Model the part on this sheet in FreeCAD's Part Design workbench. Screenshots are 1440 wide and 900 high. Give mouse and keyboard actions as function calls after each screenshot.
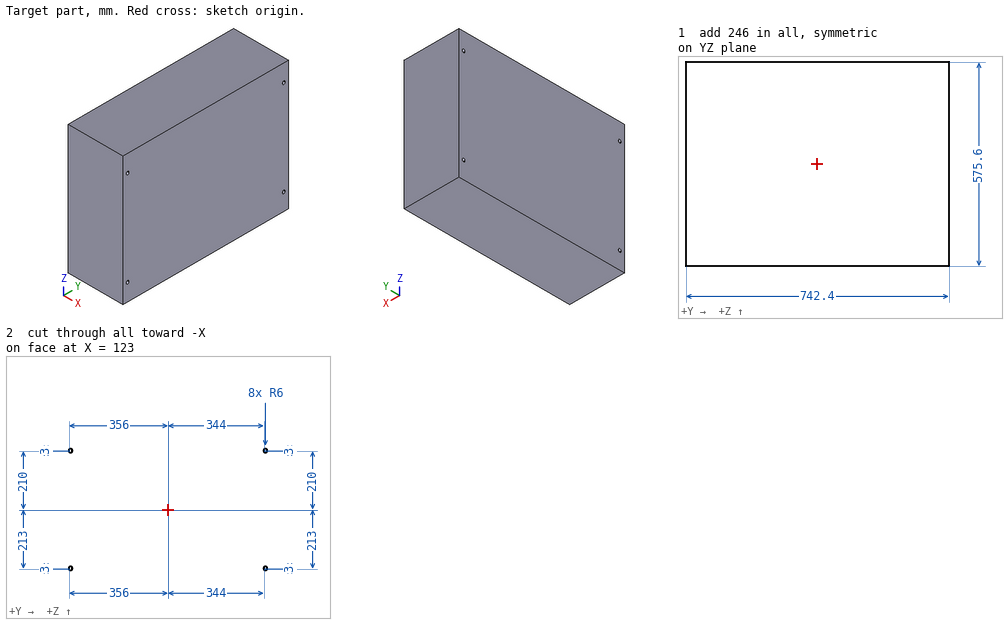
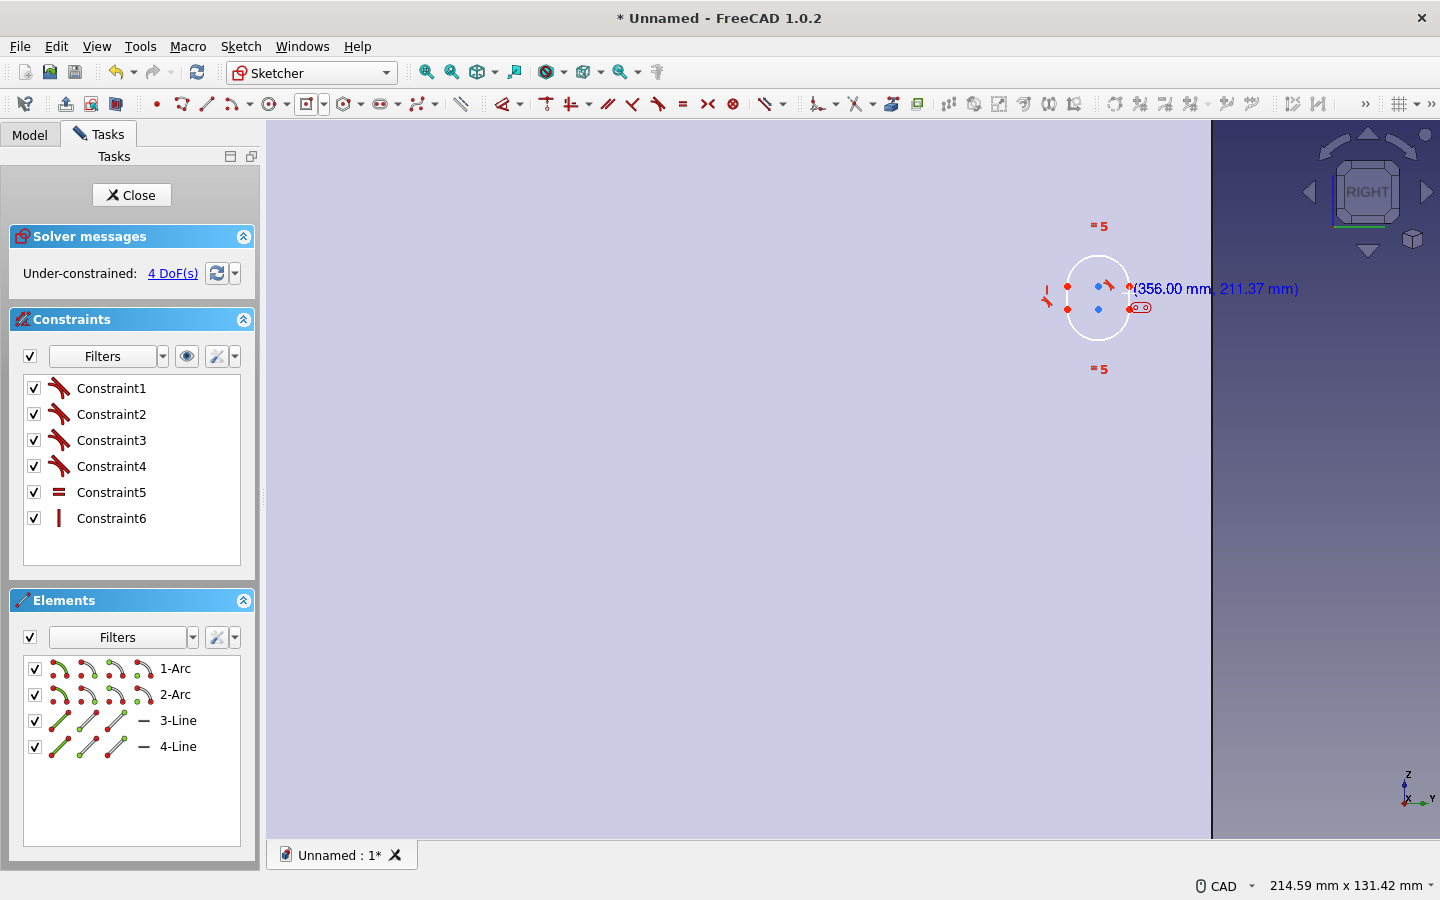
scroll(1102, 287, down, 9)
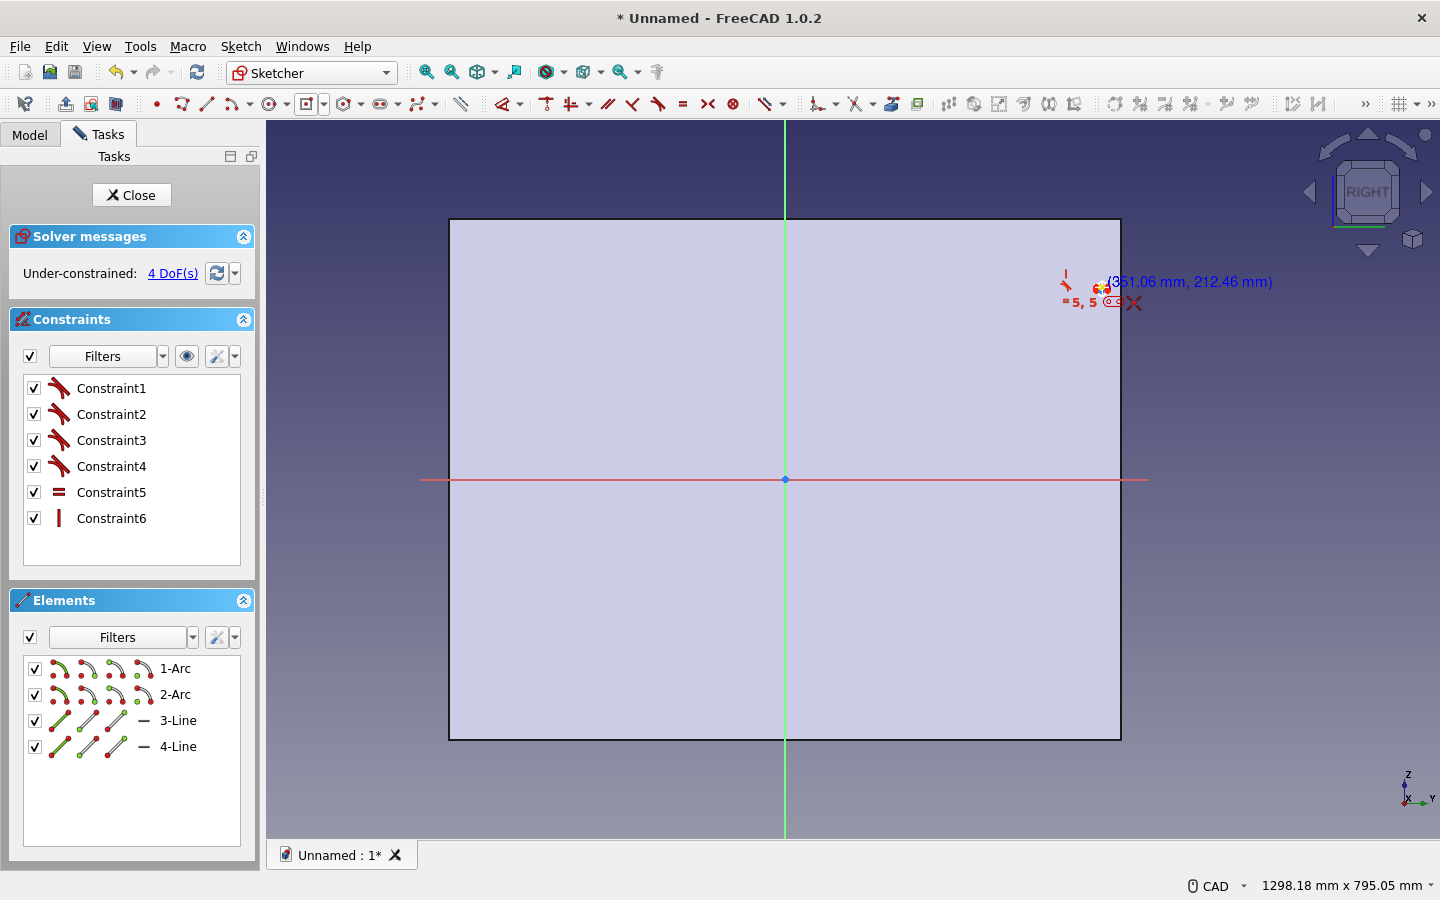
scroll(1102, 672, up, 8)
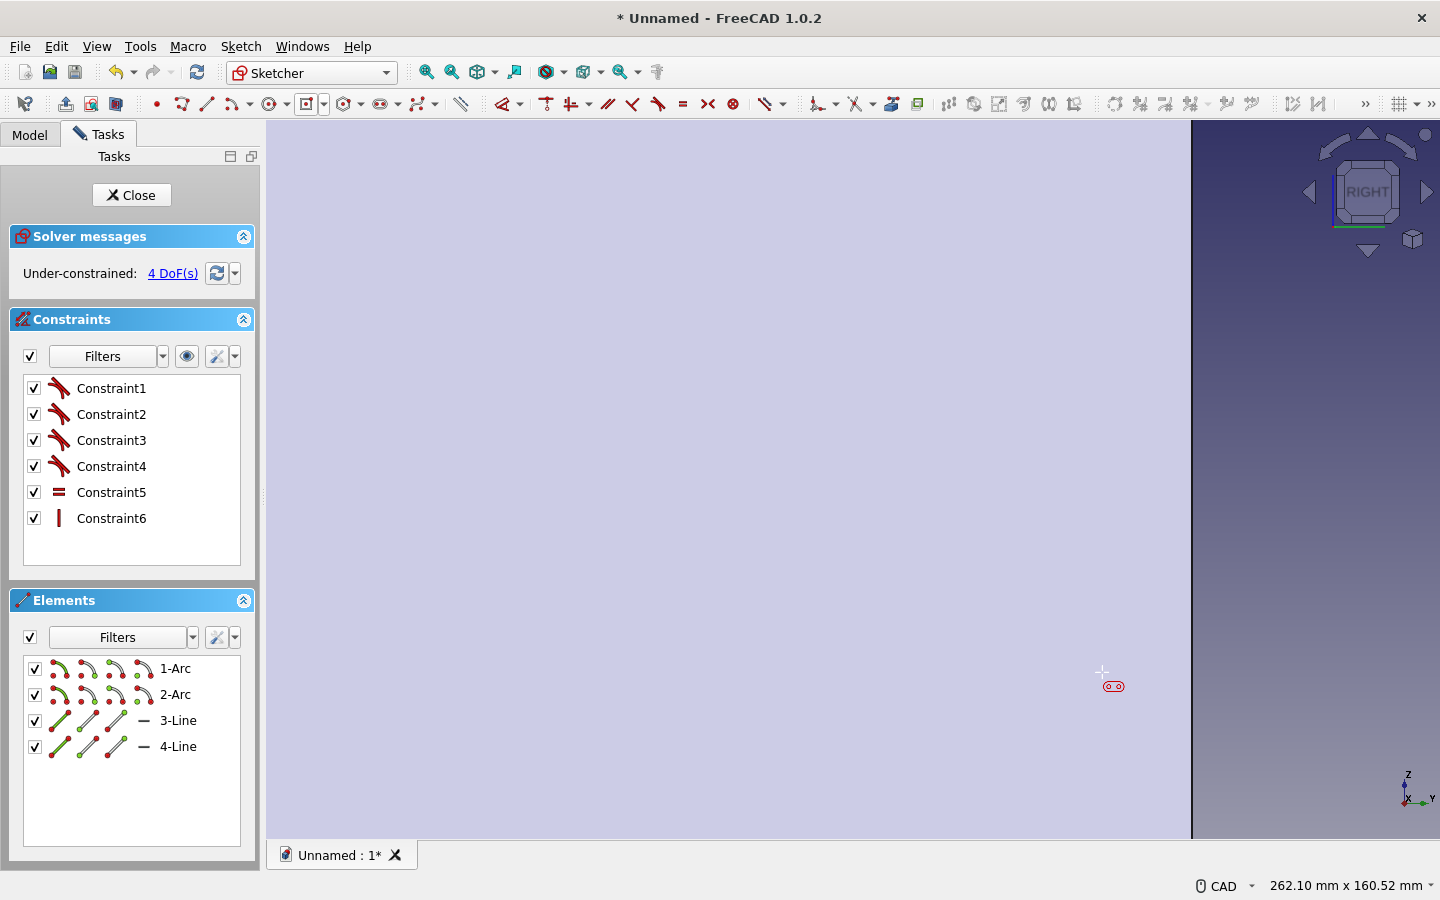
scroll(1102, 673, down, 8)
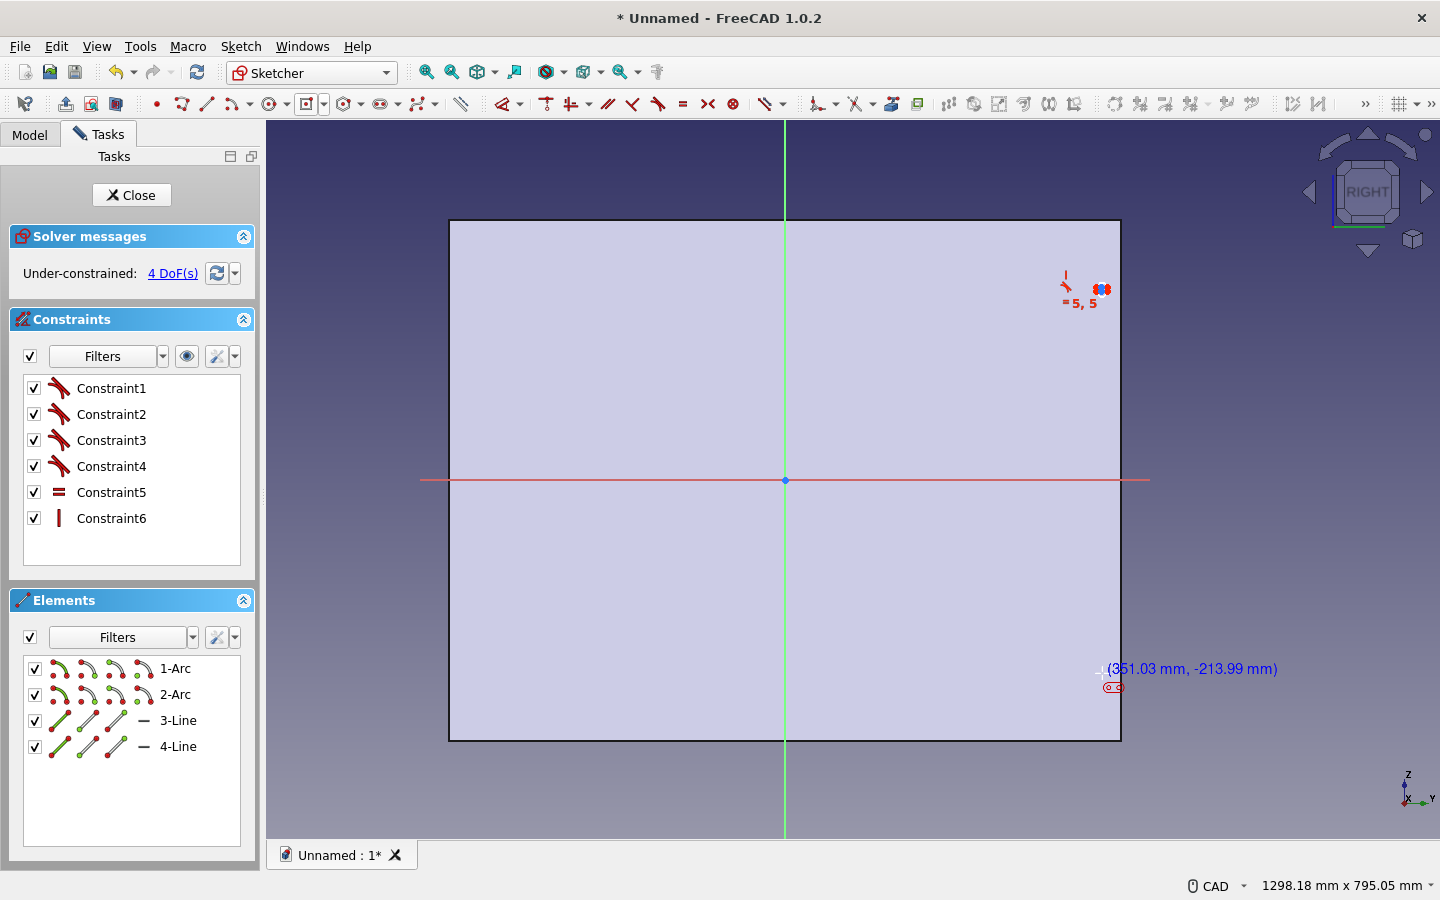
click(1102, 673)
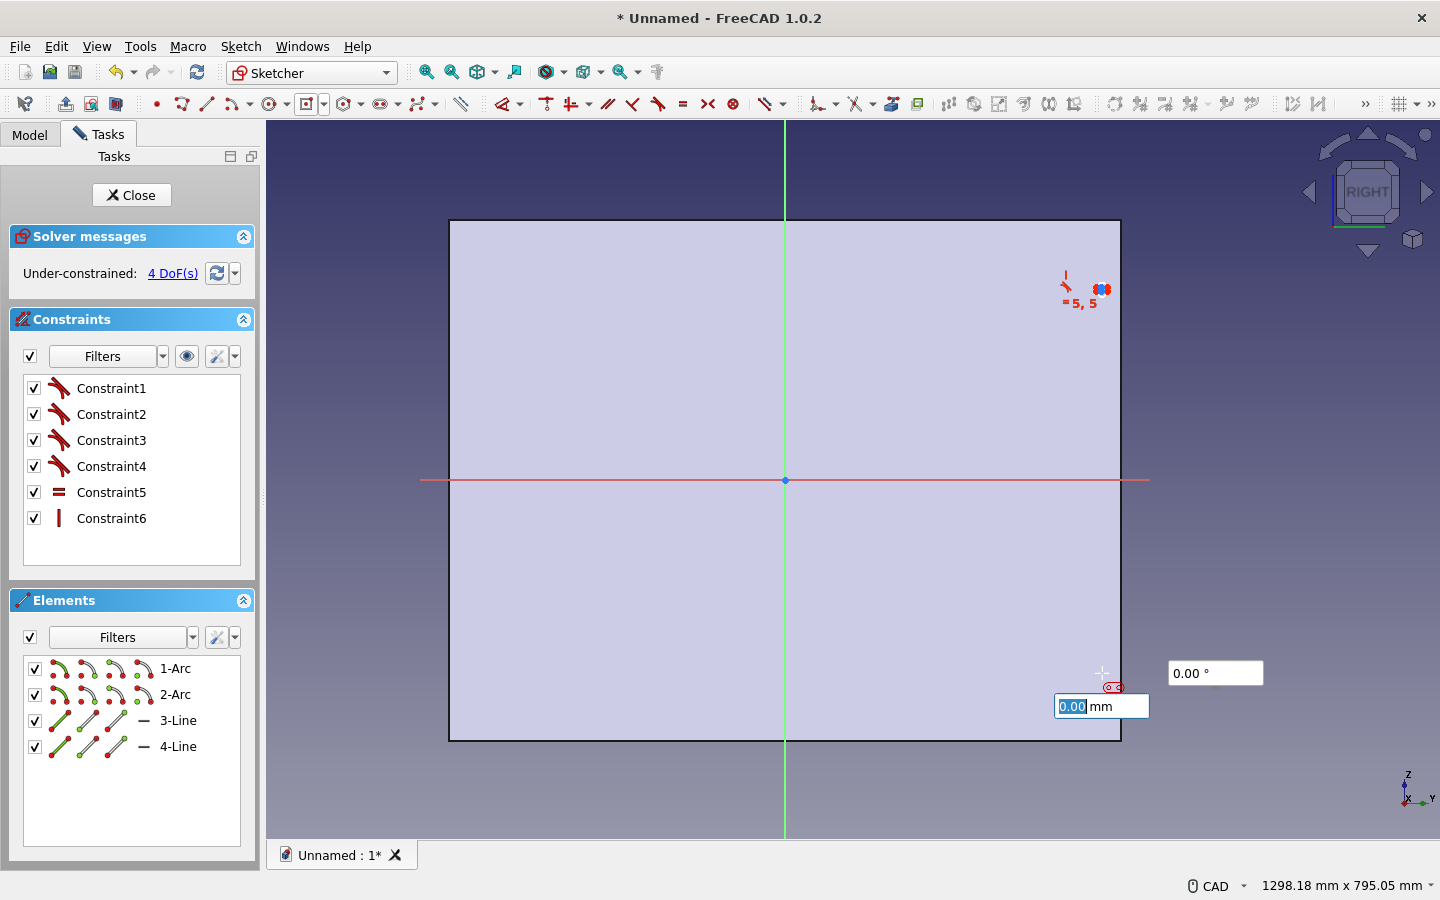
scroll(1102, 670, up, 9)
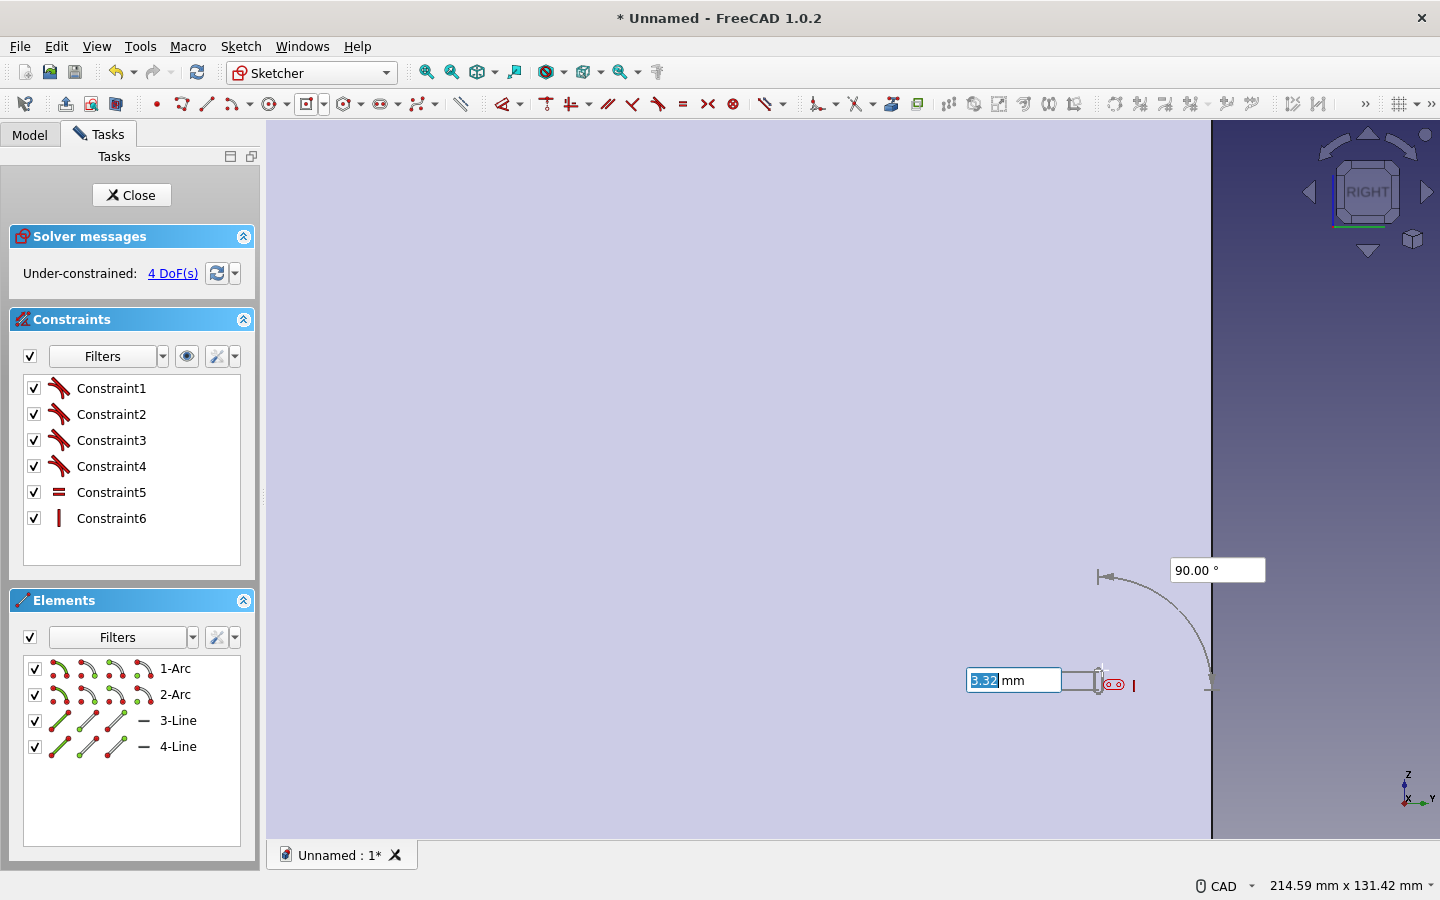
click(1098, 667)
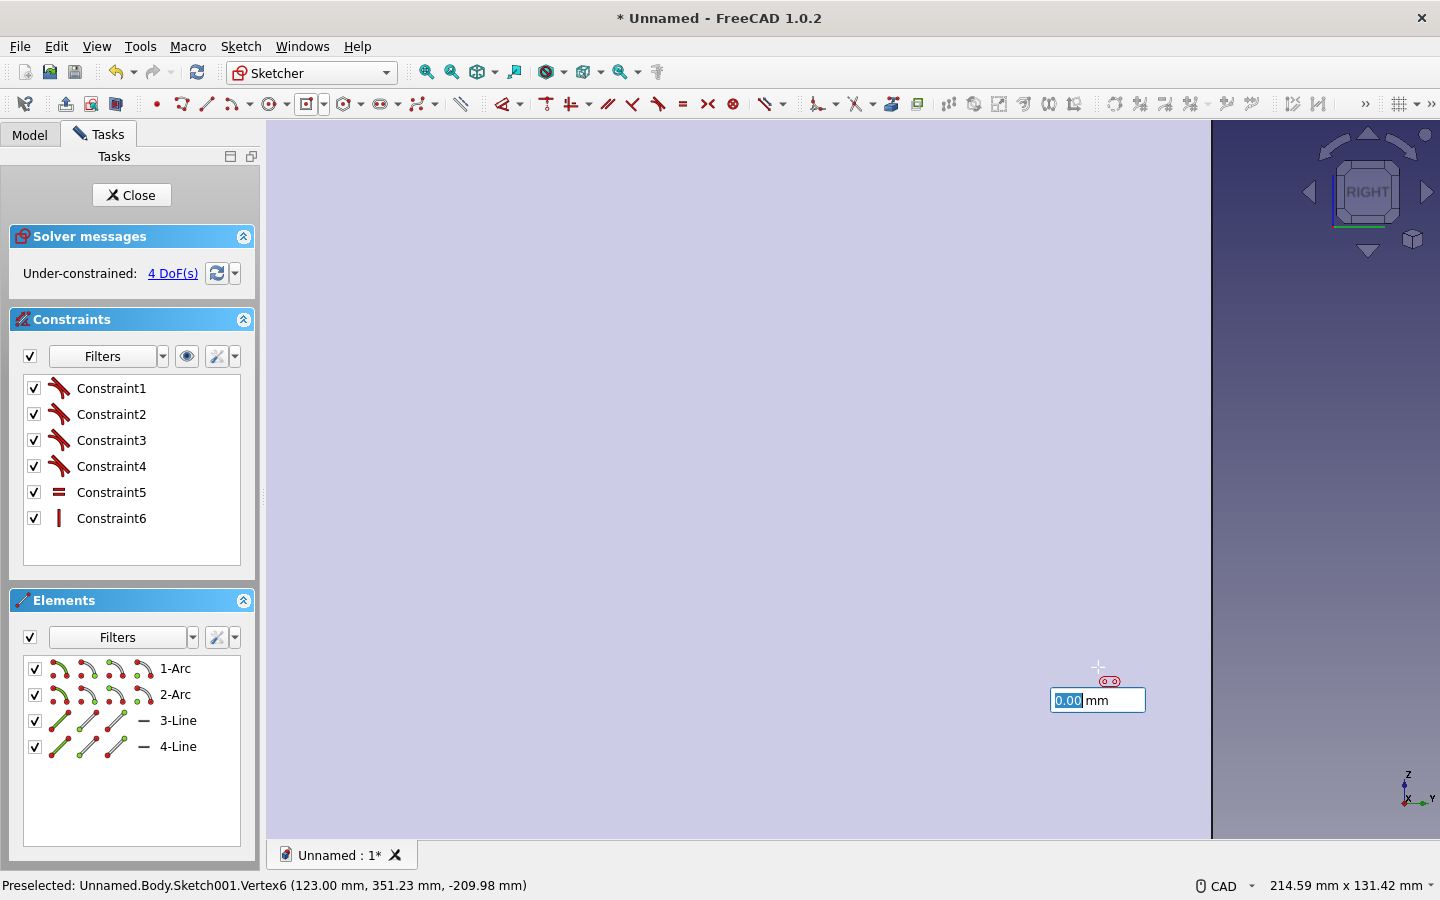
click(1129, 676)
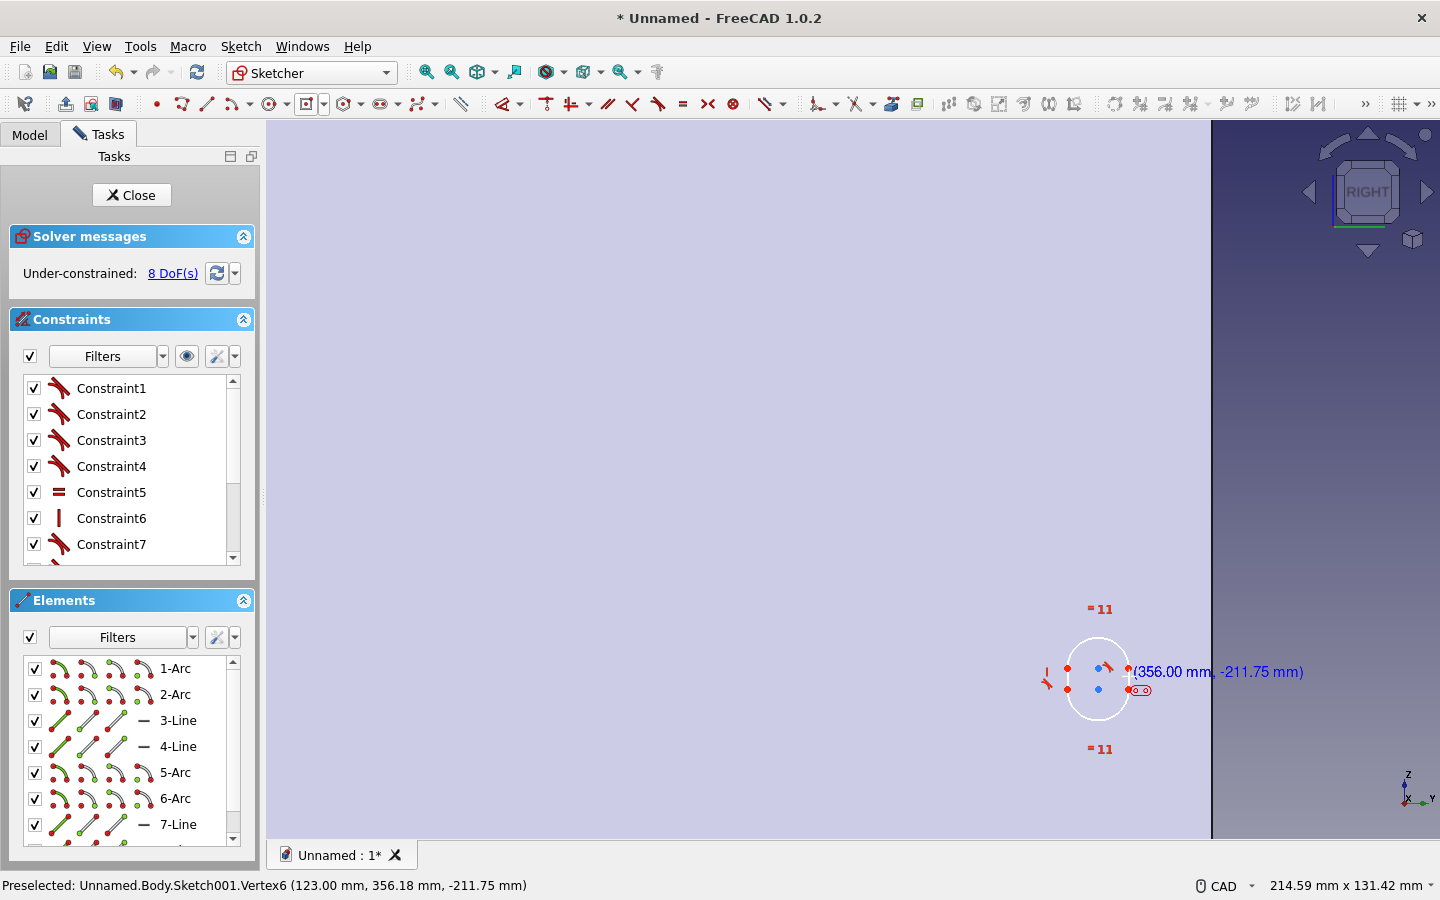
scroll(1102, 670, down, 9)